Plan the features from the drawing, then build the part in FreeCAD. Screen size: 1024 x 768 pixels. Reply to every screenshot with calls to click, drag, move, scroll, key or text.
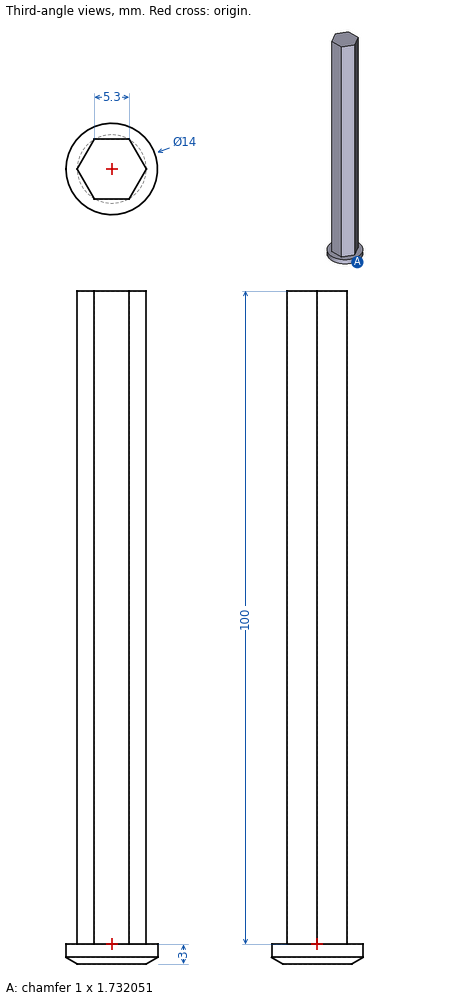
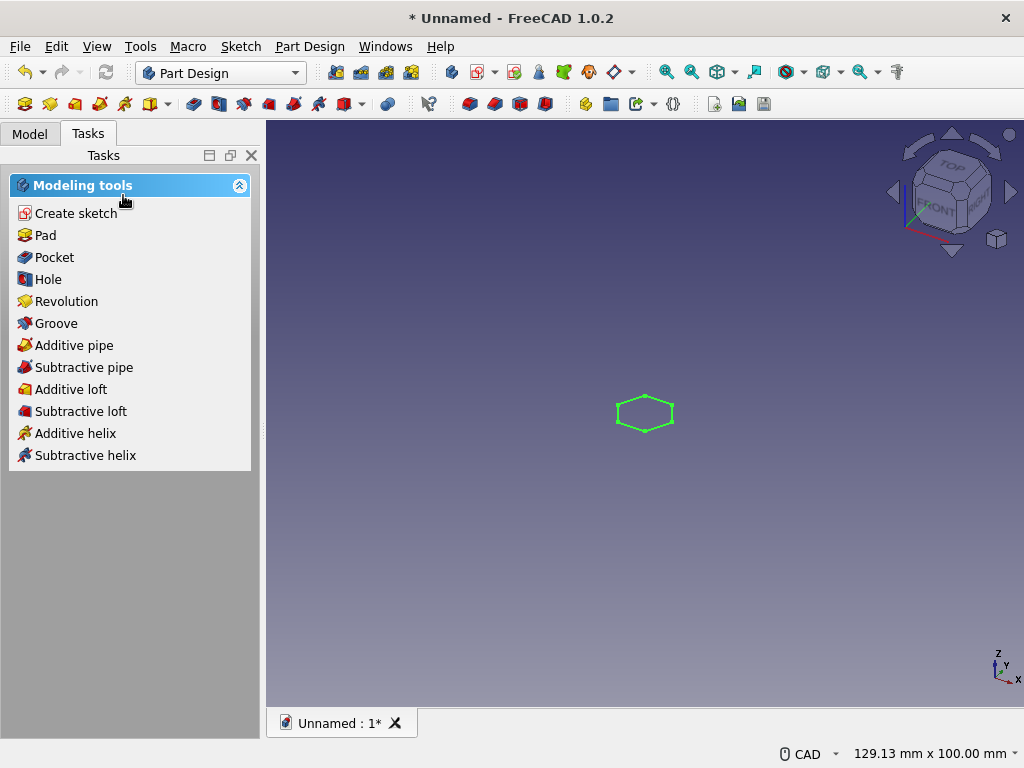
click(25, 104)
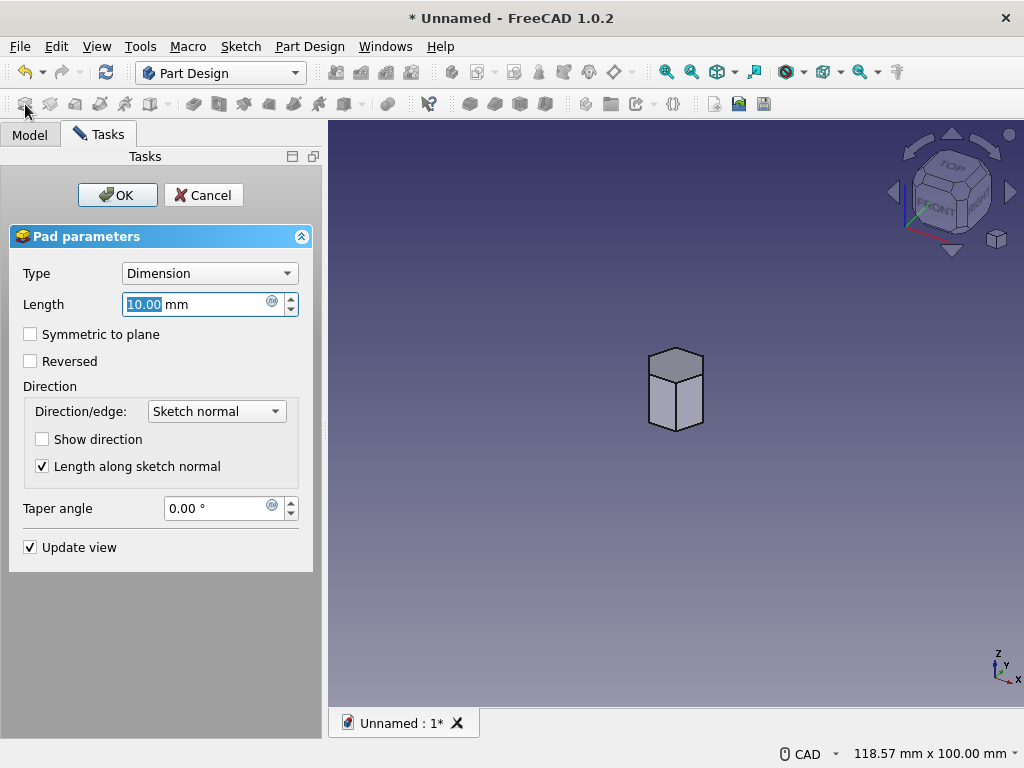
text(100)
key(Tab)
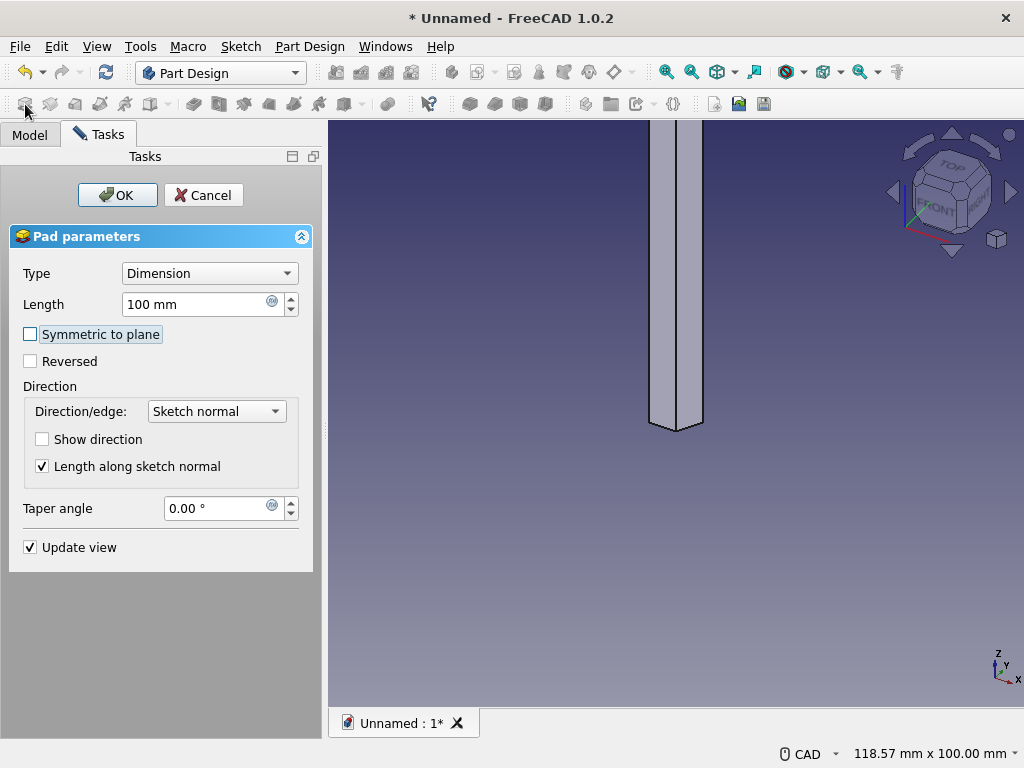
click(118, 195)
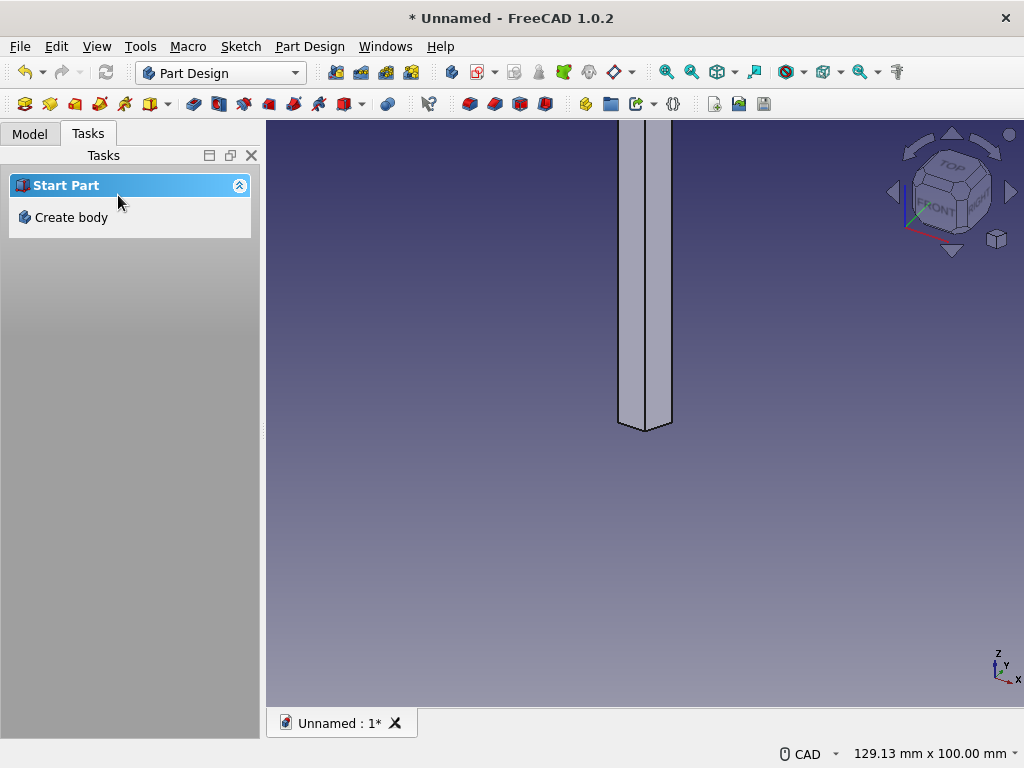
click(667, 72)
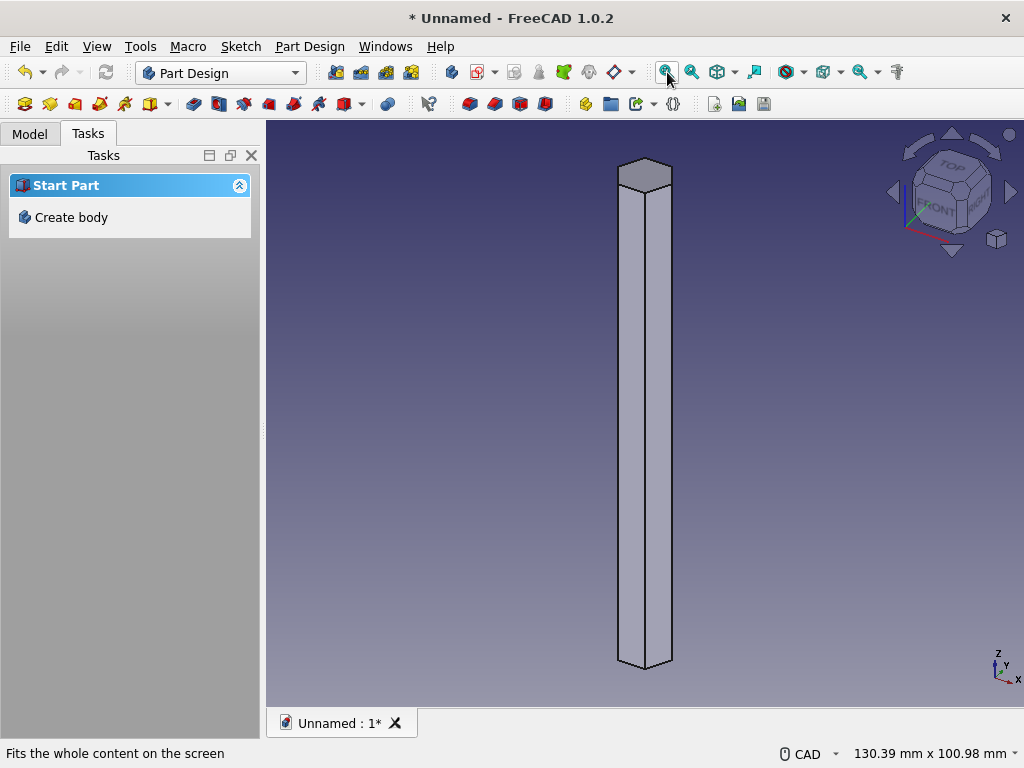
click(476, 72)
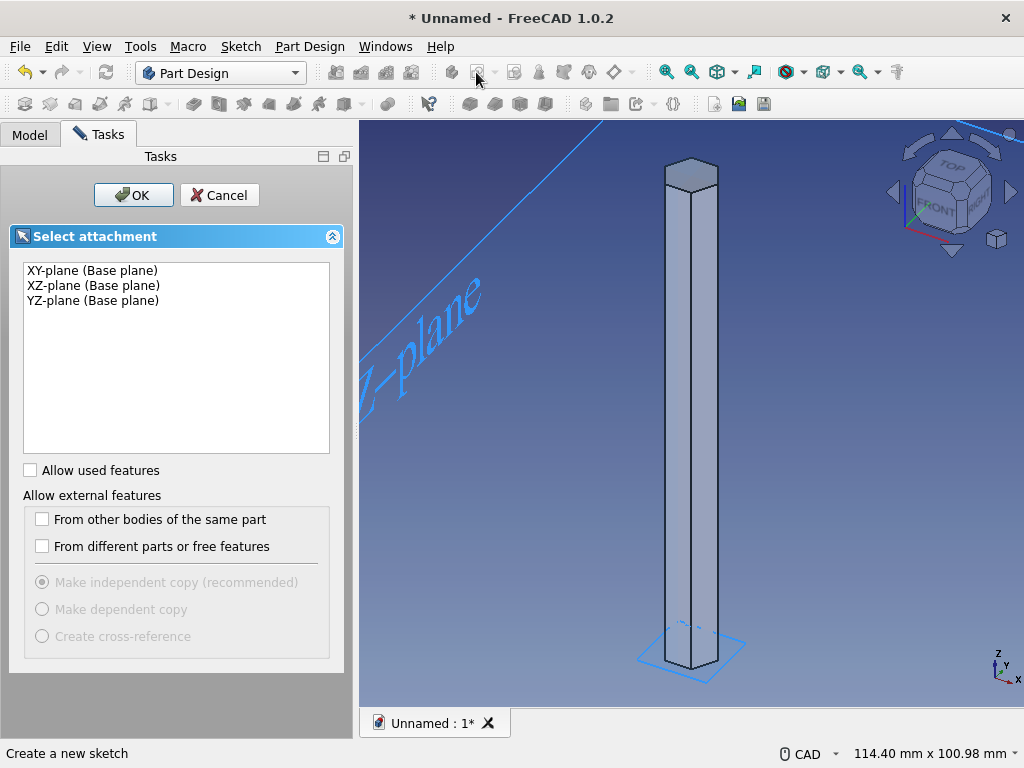
click(84, 270)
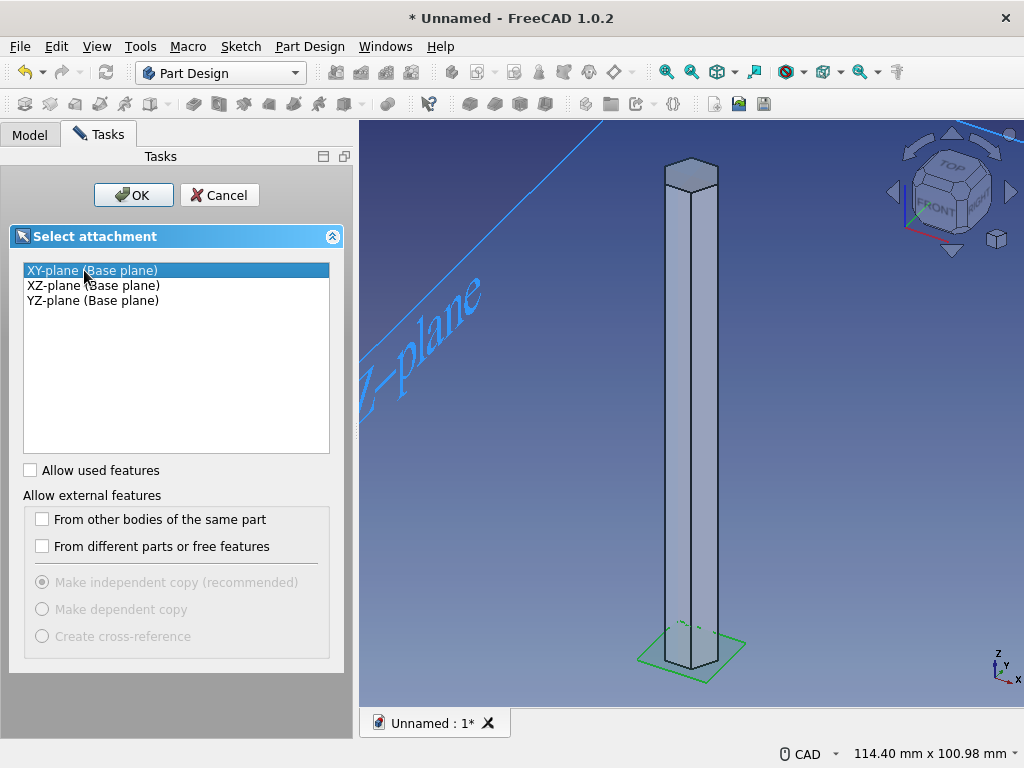
click(134, 195)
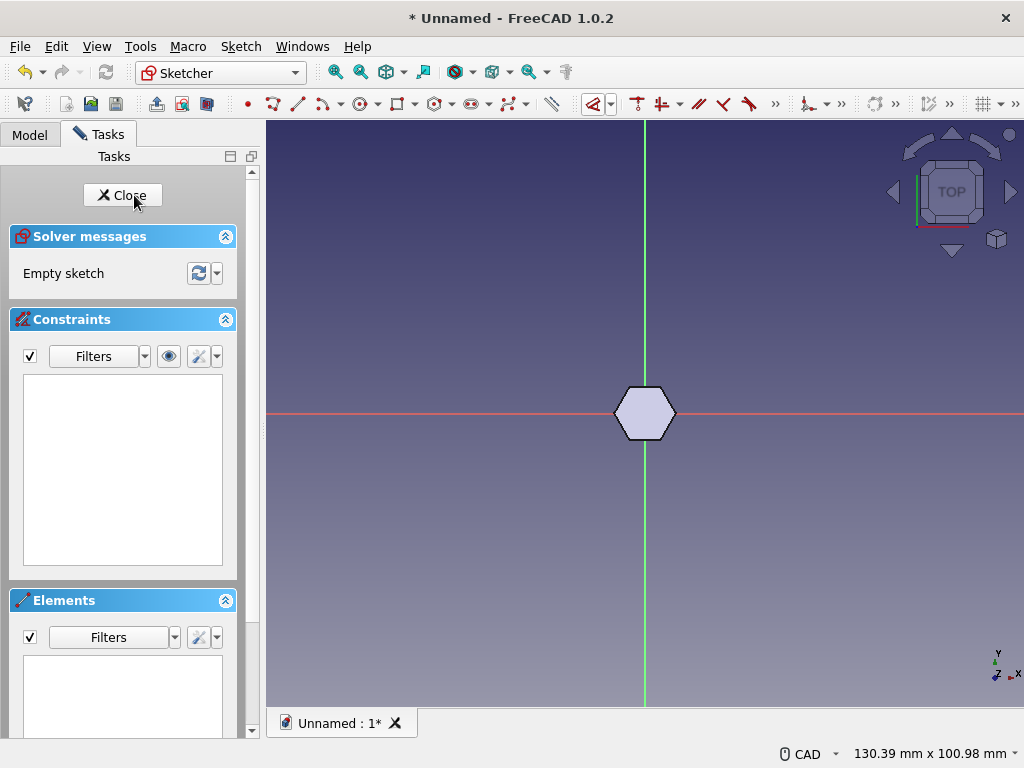
click(207, 104)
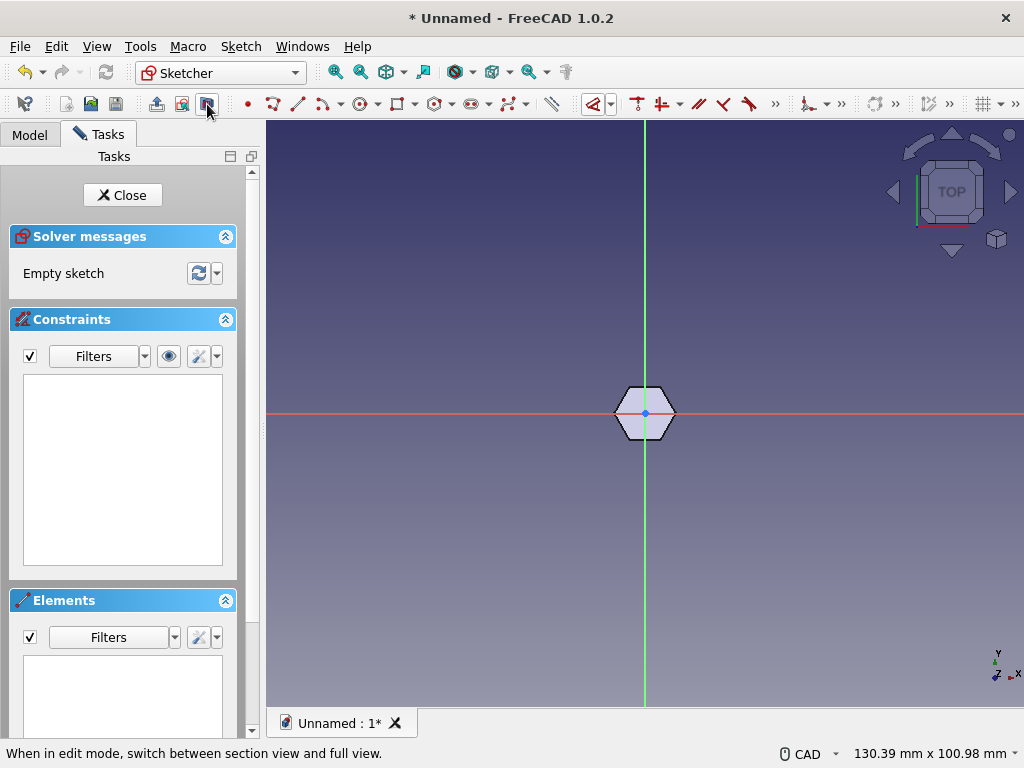
scroll(662, 414, up, 8)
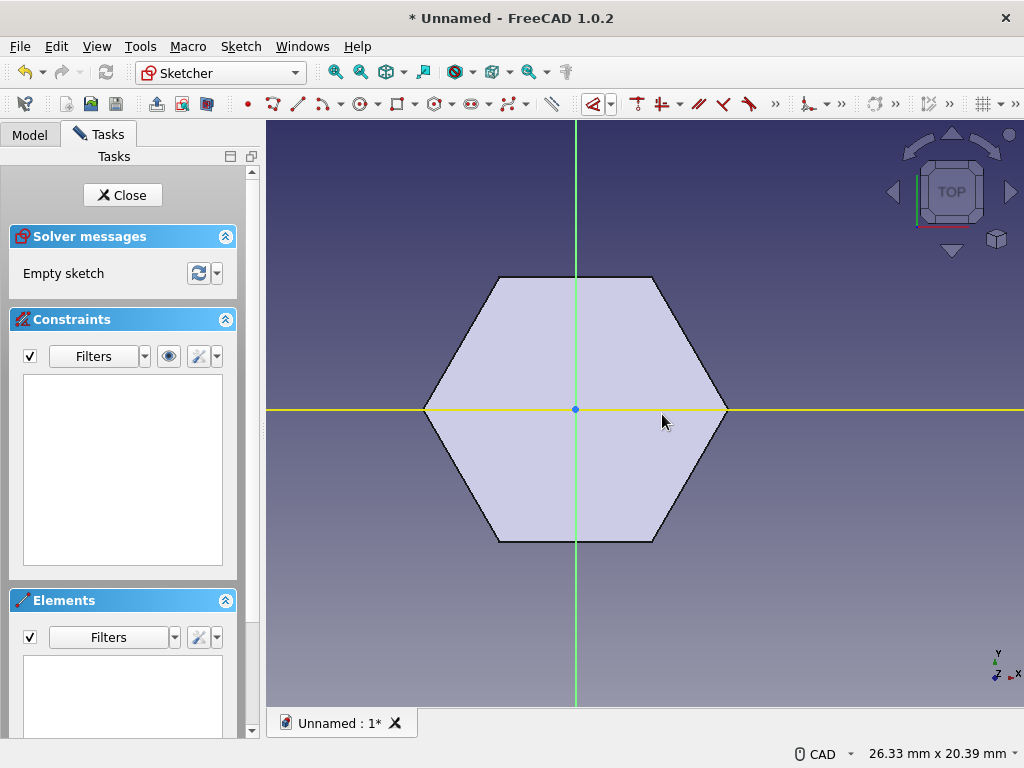
click(360, 104)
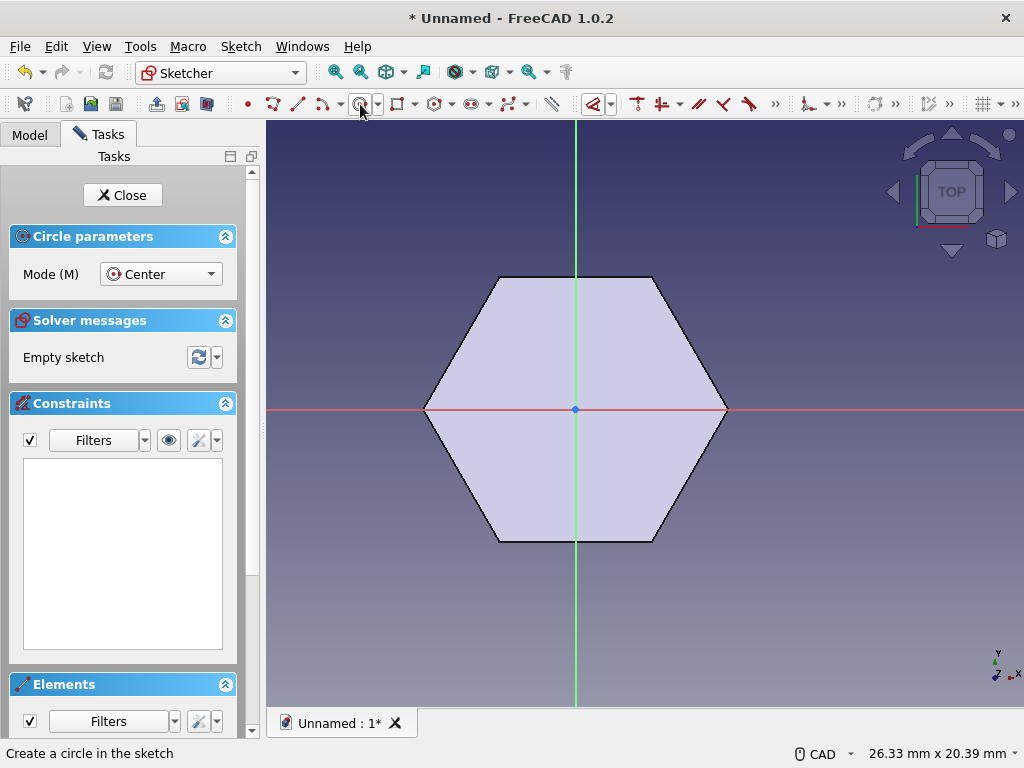
click(576, 410)
move(718, 267)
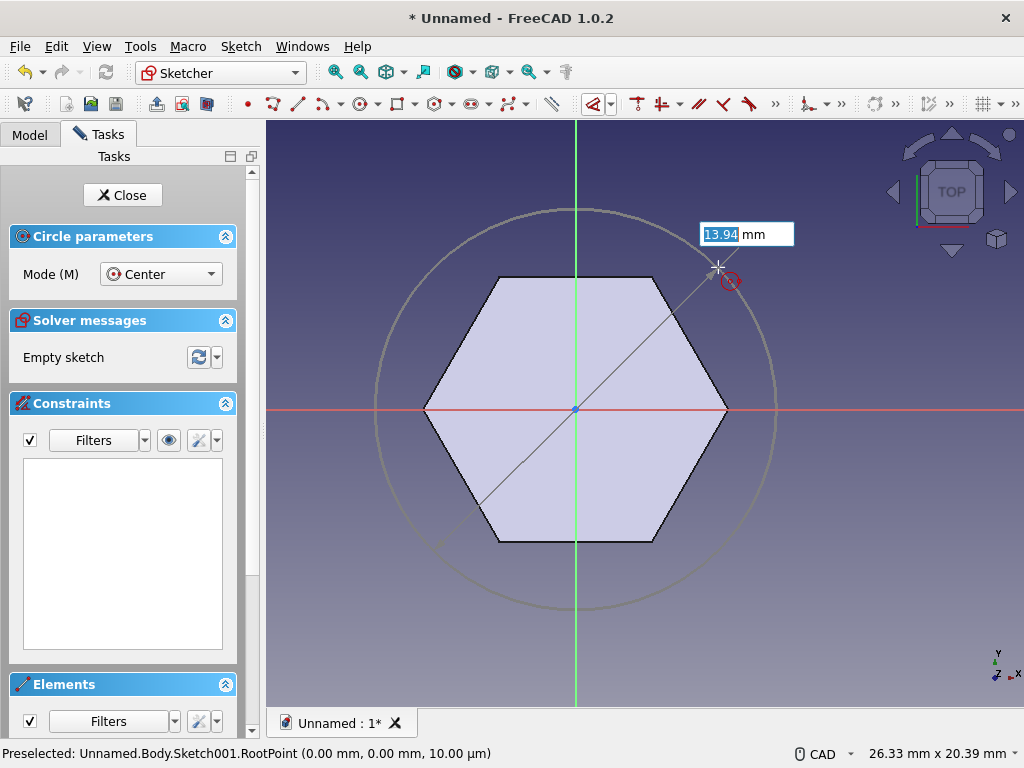
text(14)
key(Return)
key(Escape)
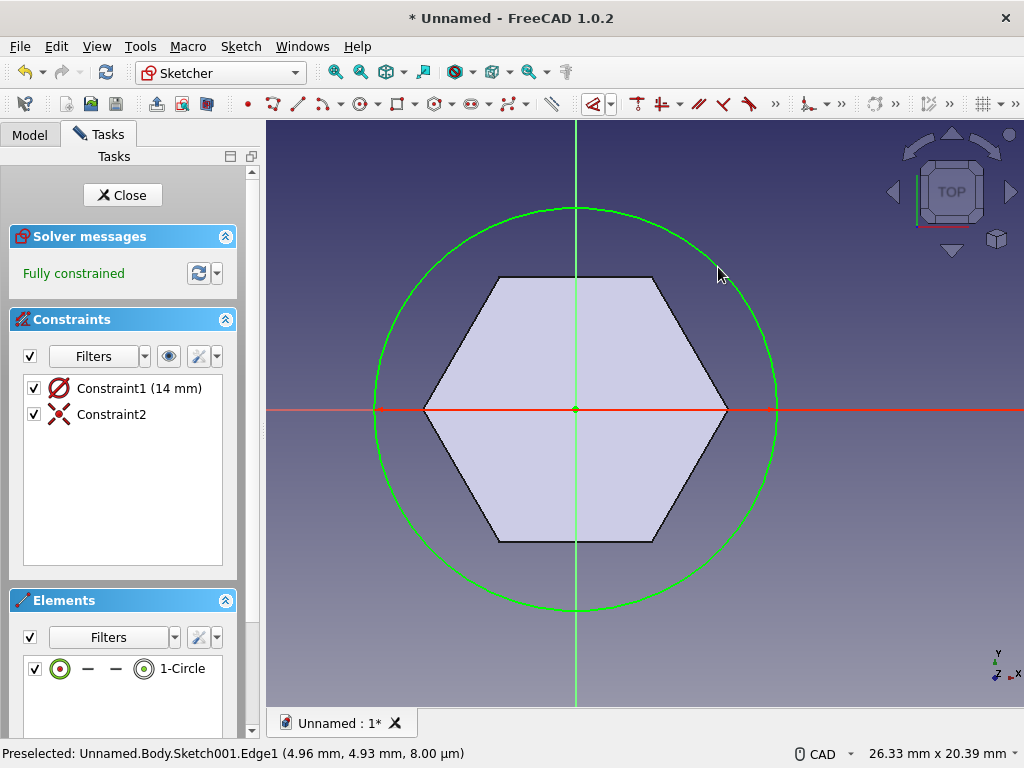
click(123, 195)